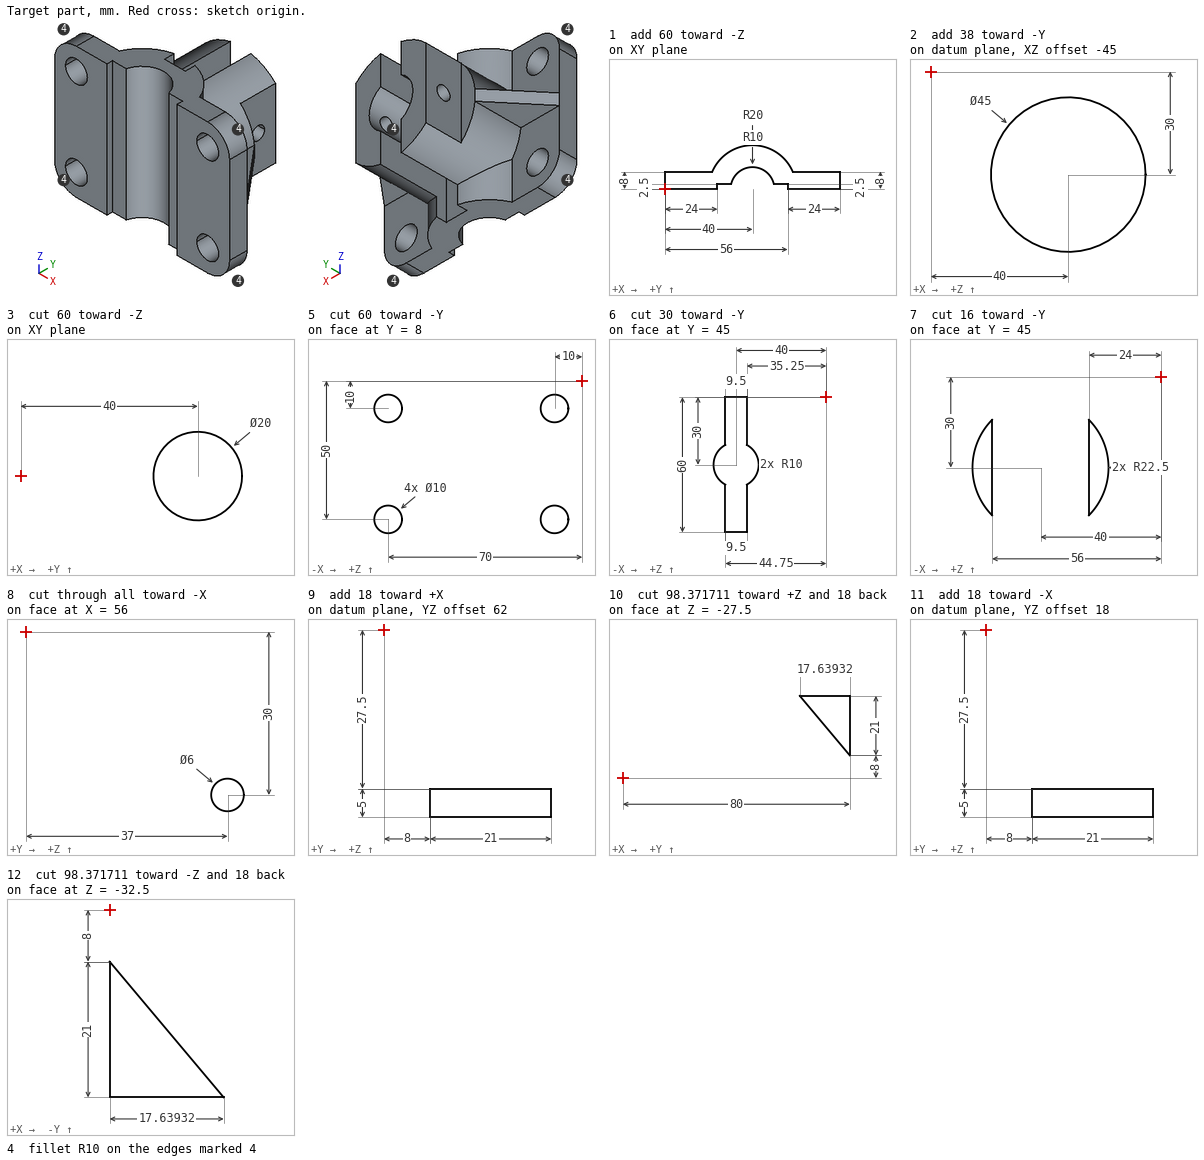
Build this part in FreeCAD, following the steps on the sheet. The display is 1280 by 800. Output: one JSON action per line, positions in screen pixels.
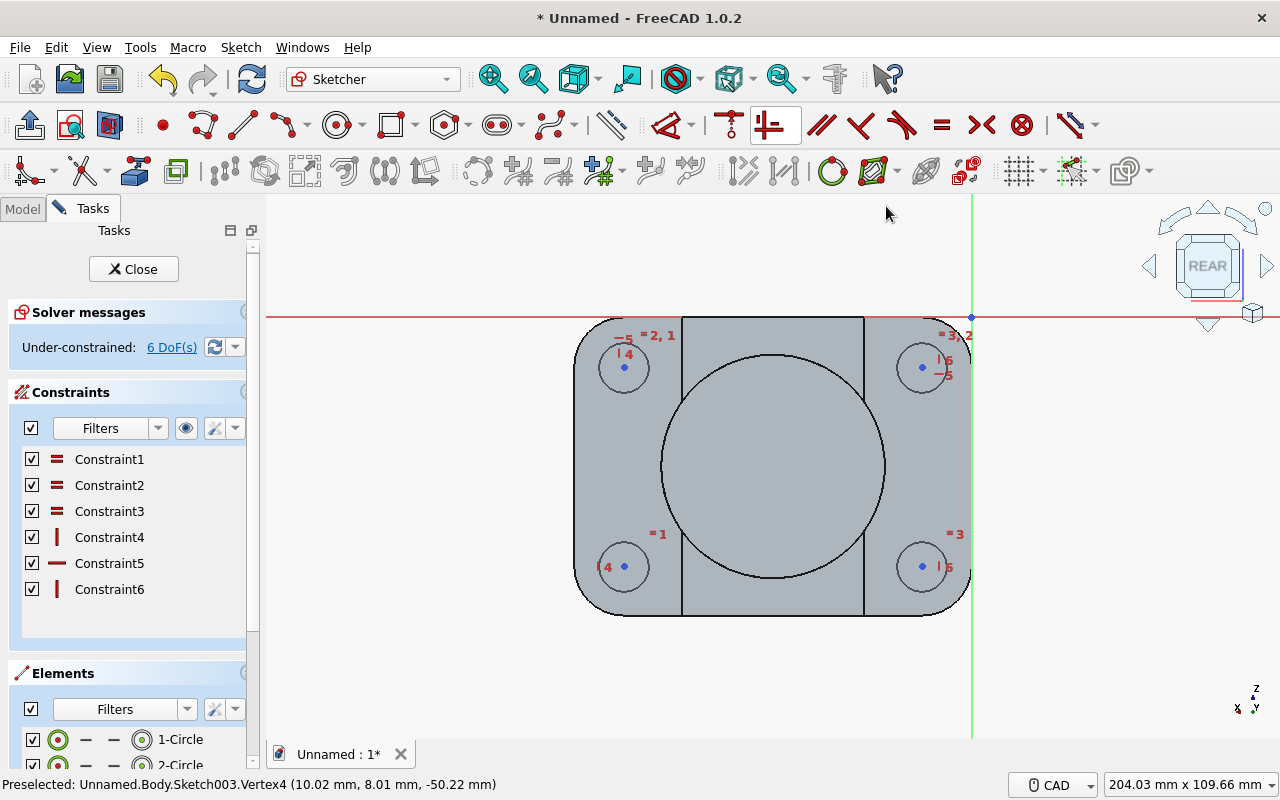
{"action": "left_click", "coordinate": [624, 567]}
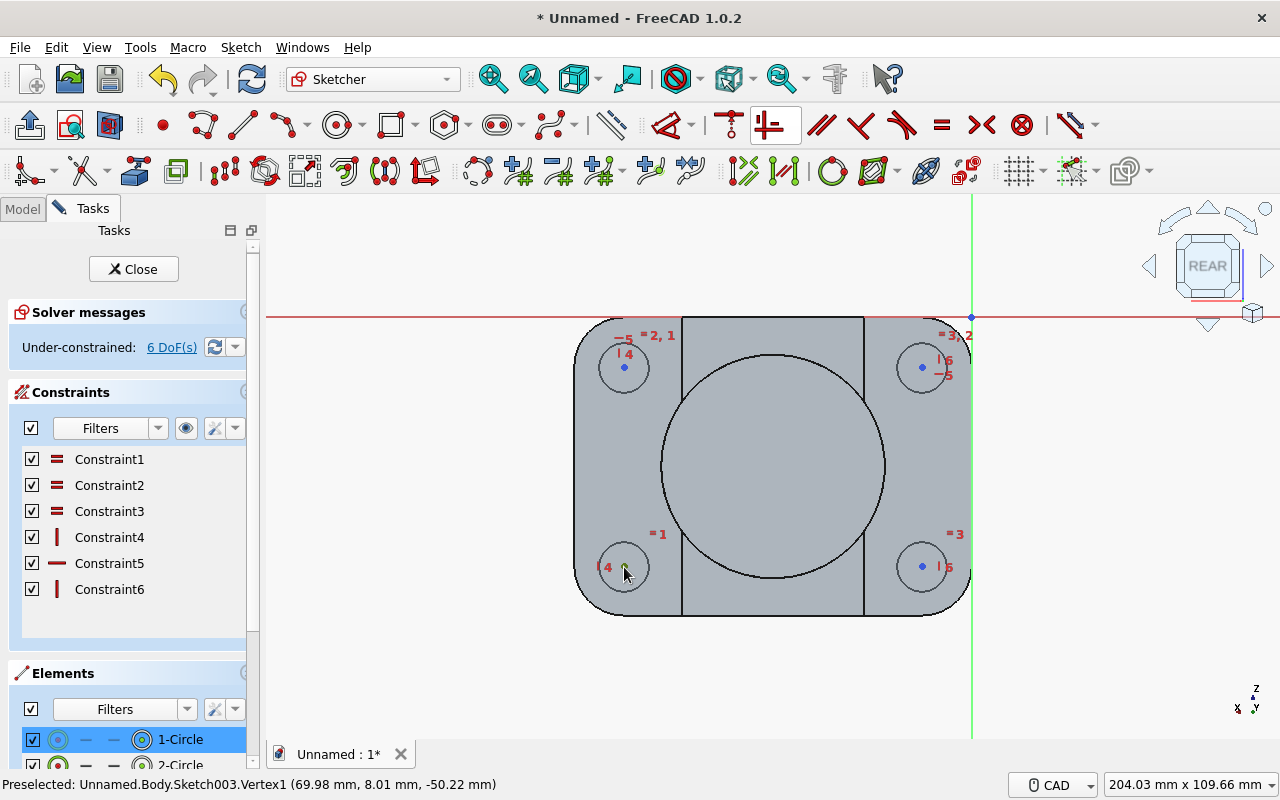
{"action": "left_click", "coordinate": [922, 567]}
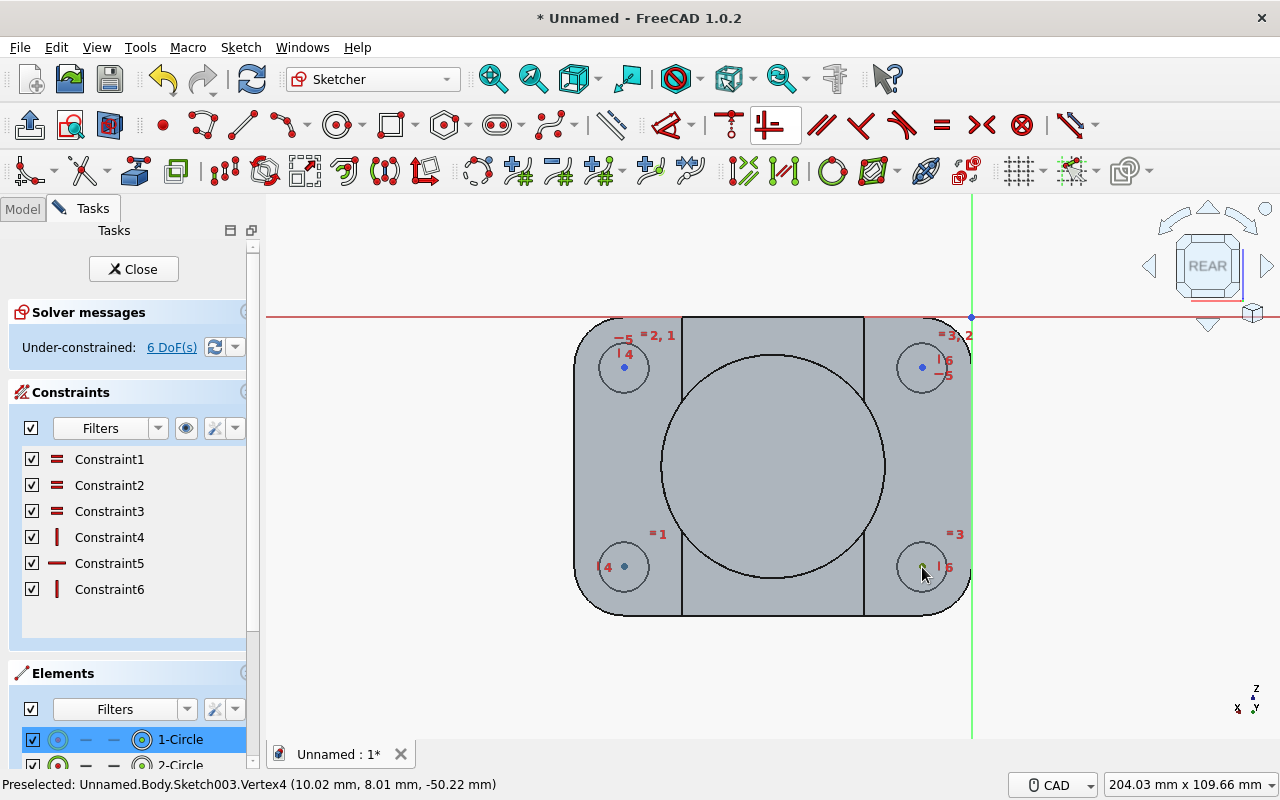
{"action": "key", "text": "h"}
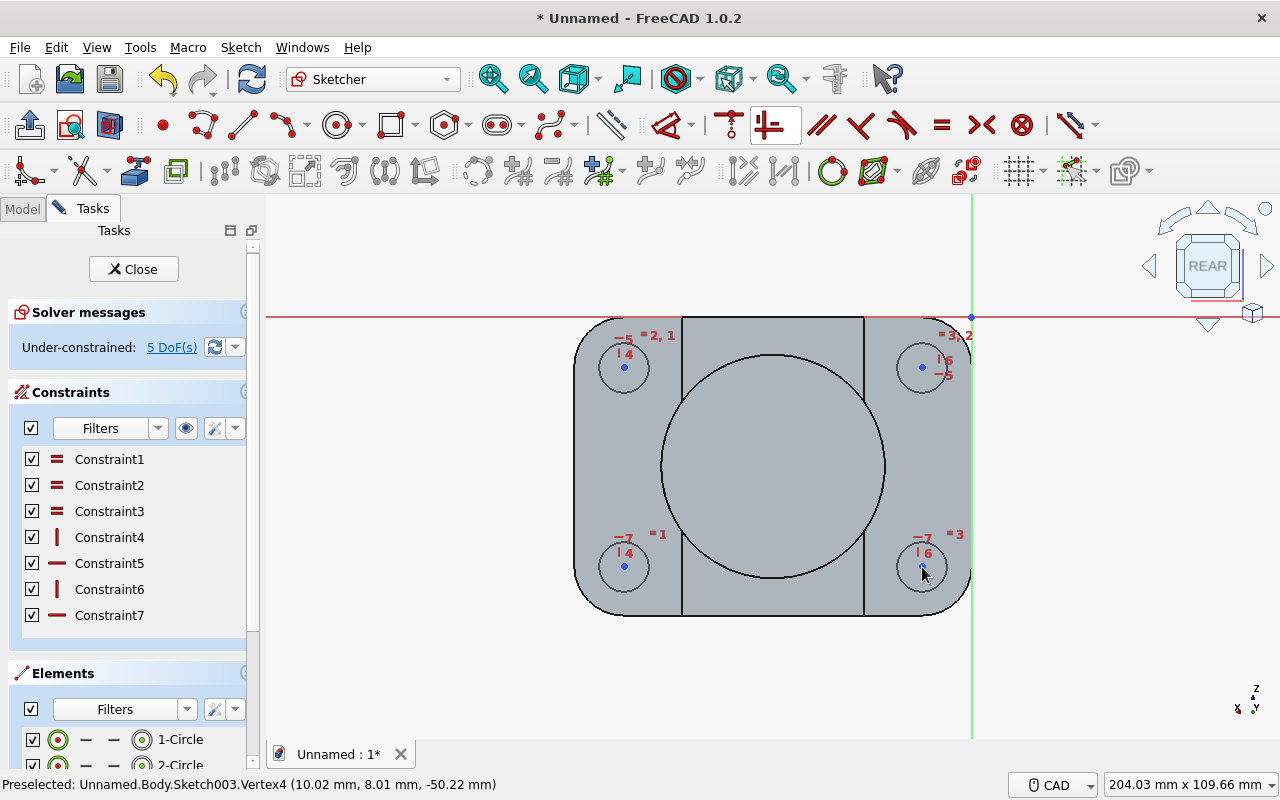
{"action": "left_click", "coordinate": [666, 126]}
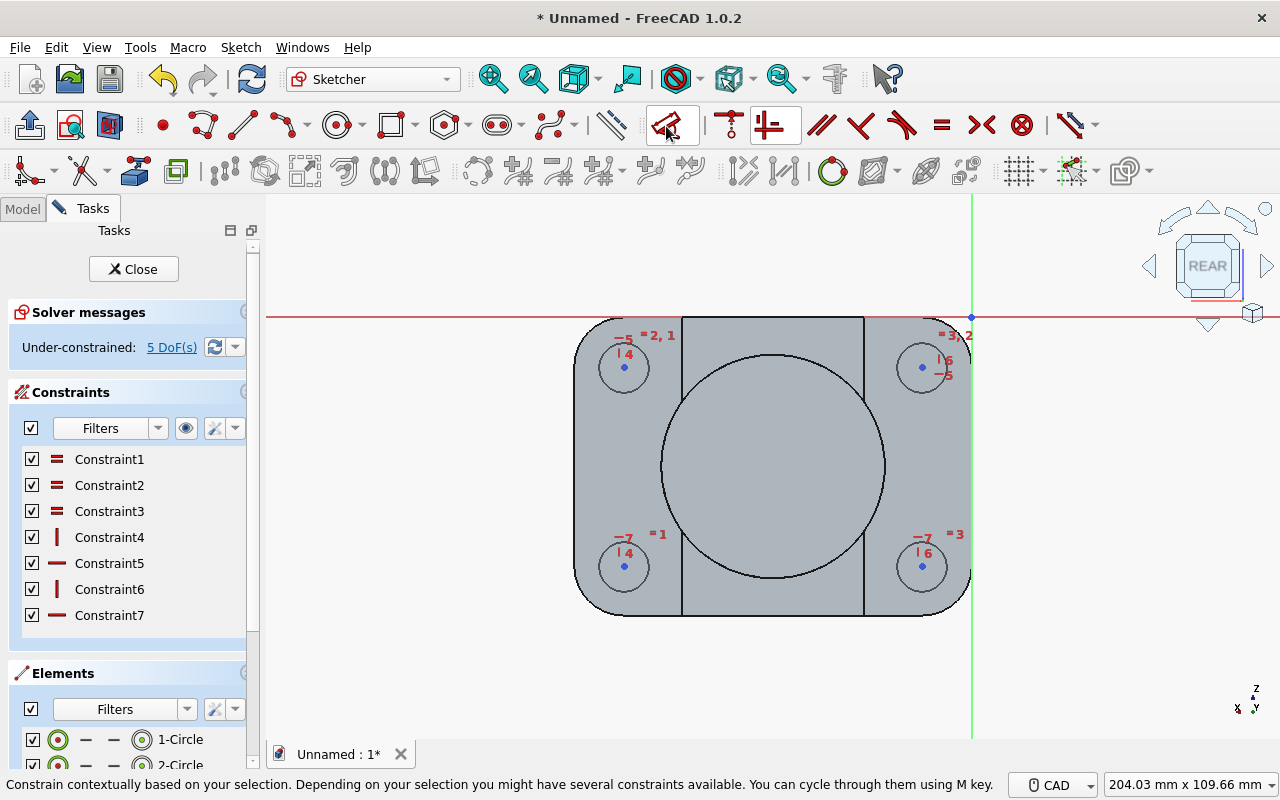
{"action": "left_click", "coordinate": [641, 549]}
{"action": "left_click", "coordinate": [663, 526]}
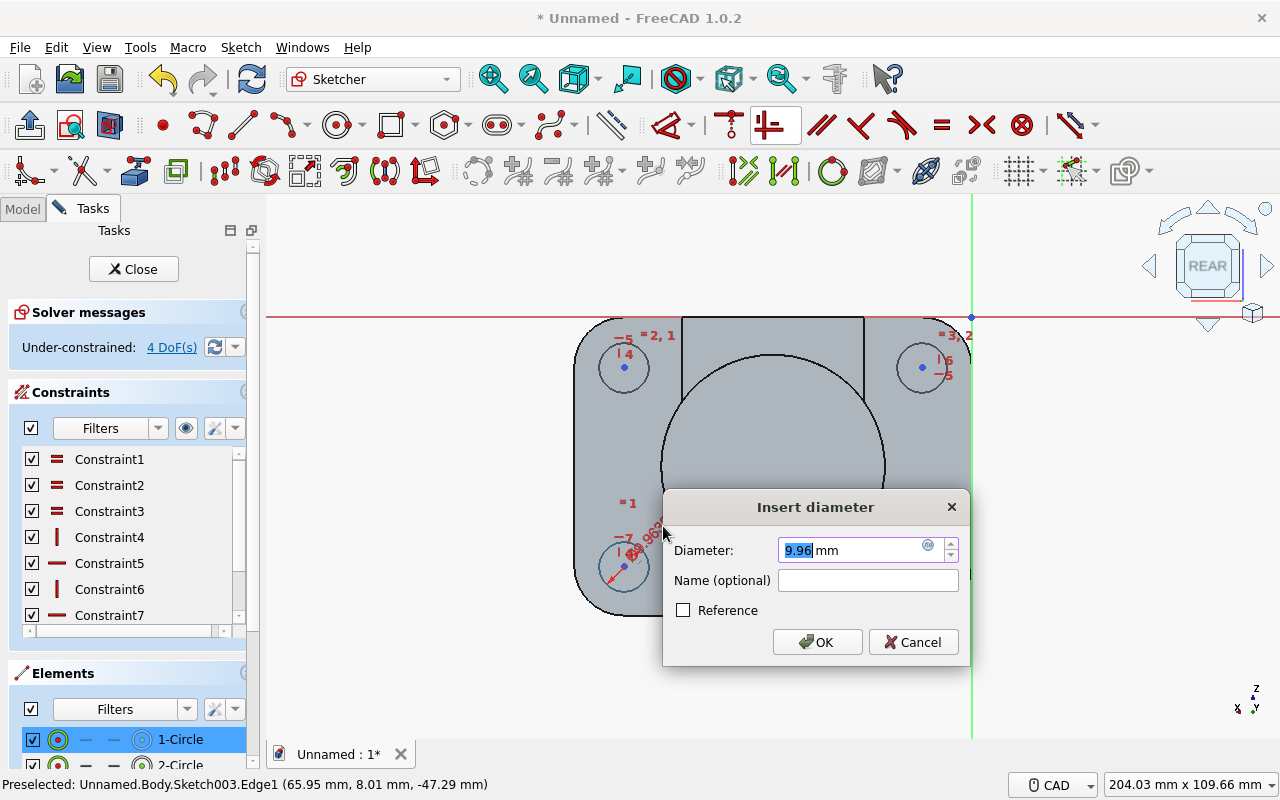
{"action": "type", "text": "10"}
{"action": "key", "text": "Return"}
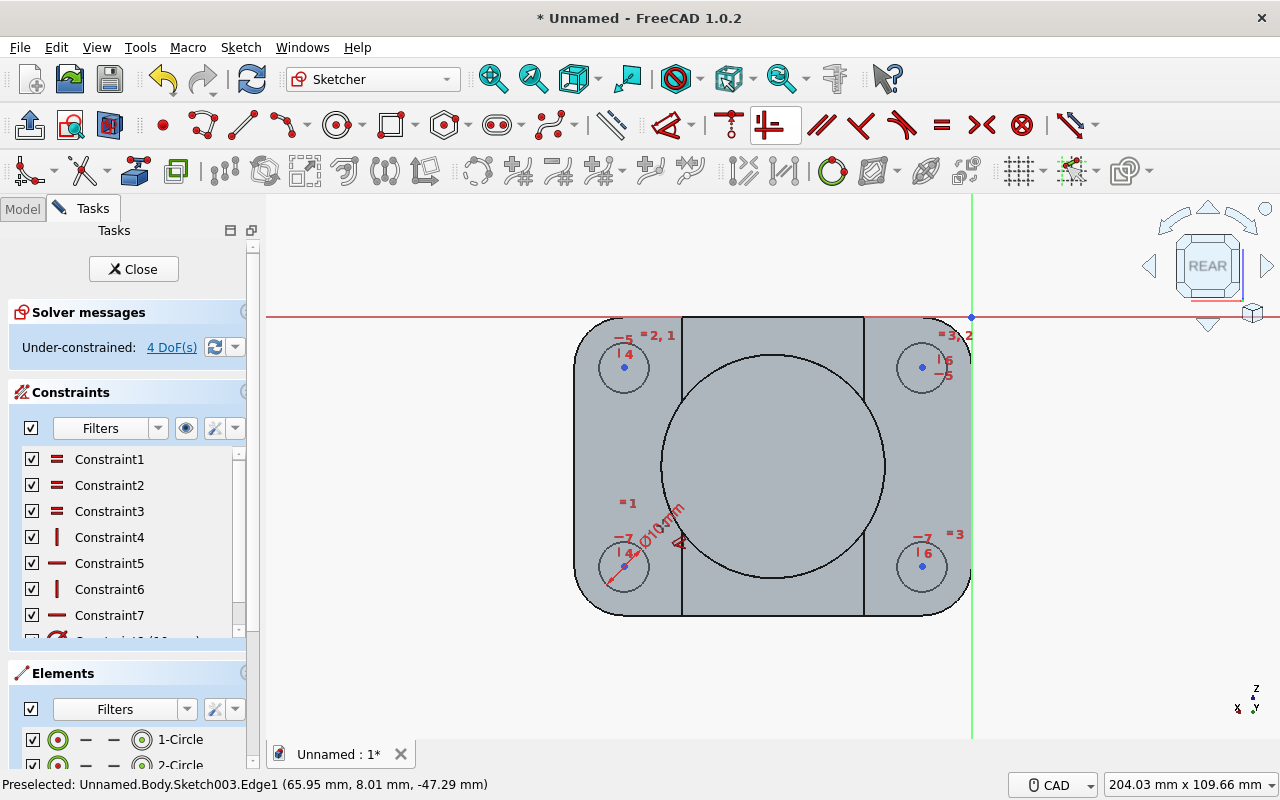
{"action": "left_click", "coordinate": [624, 567]}
{"action": "left_click", "coordinate": [798, 283]}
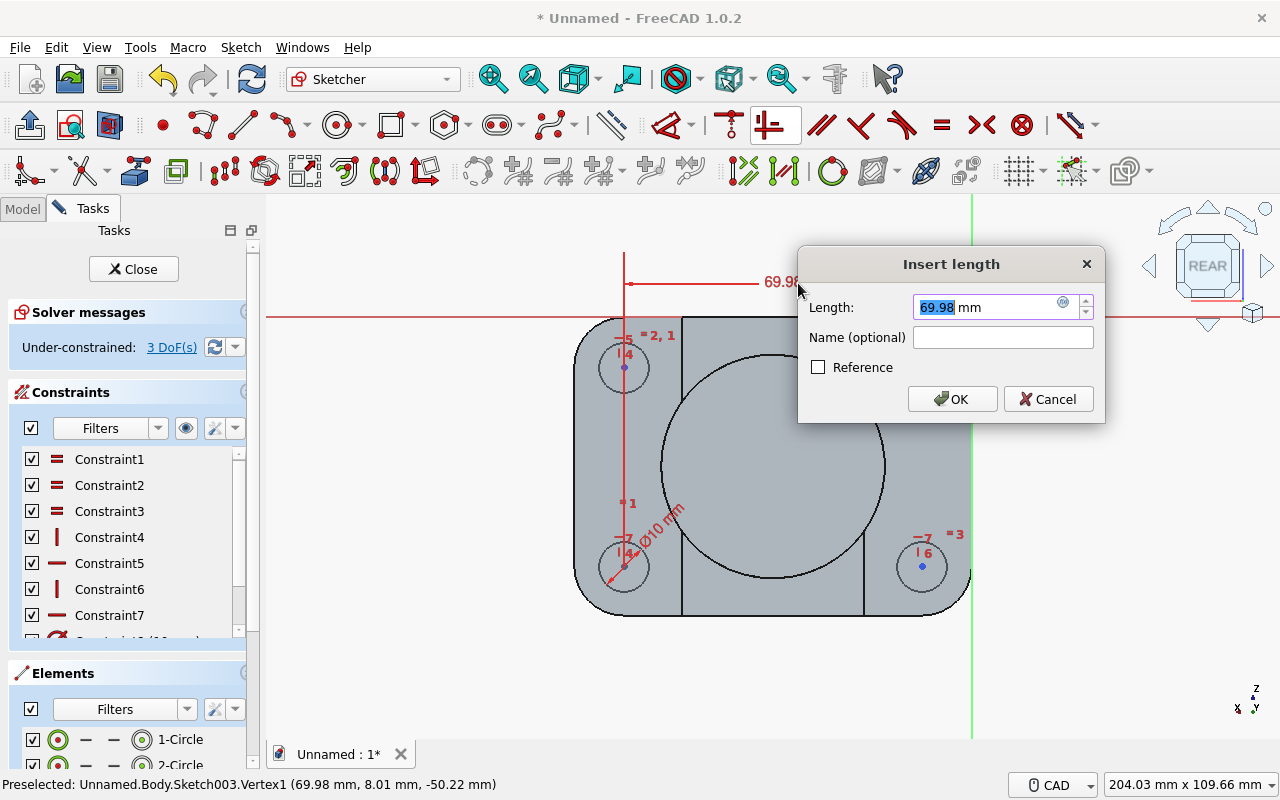
{"action": "type", "text": "70"}
{"action": "key", "text": "Return"}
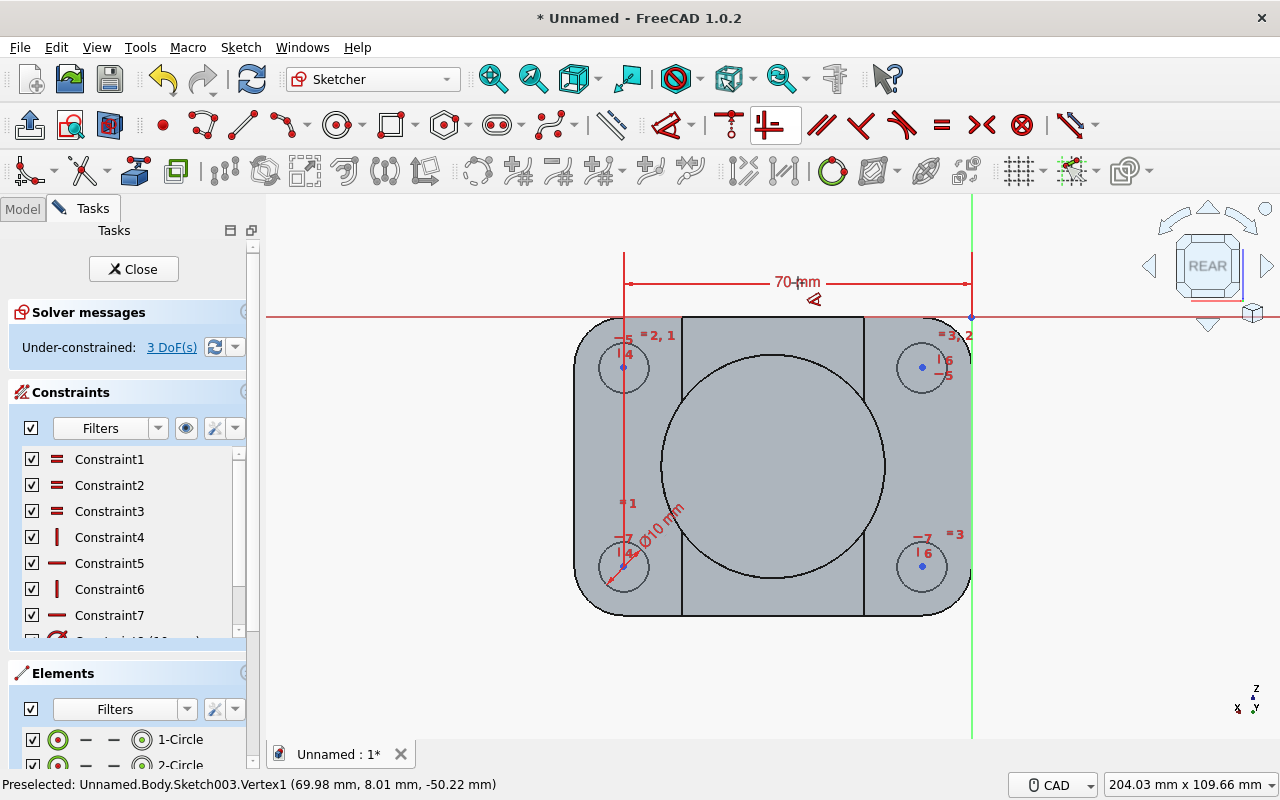
{"action": "left_click", "coordinate": [624, 567]}
{"action": "left_click", "coordinate": [1006, 442]}